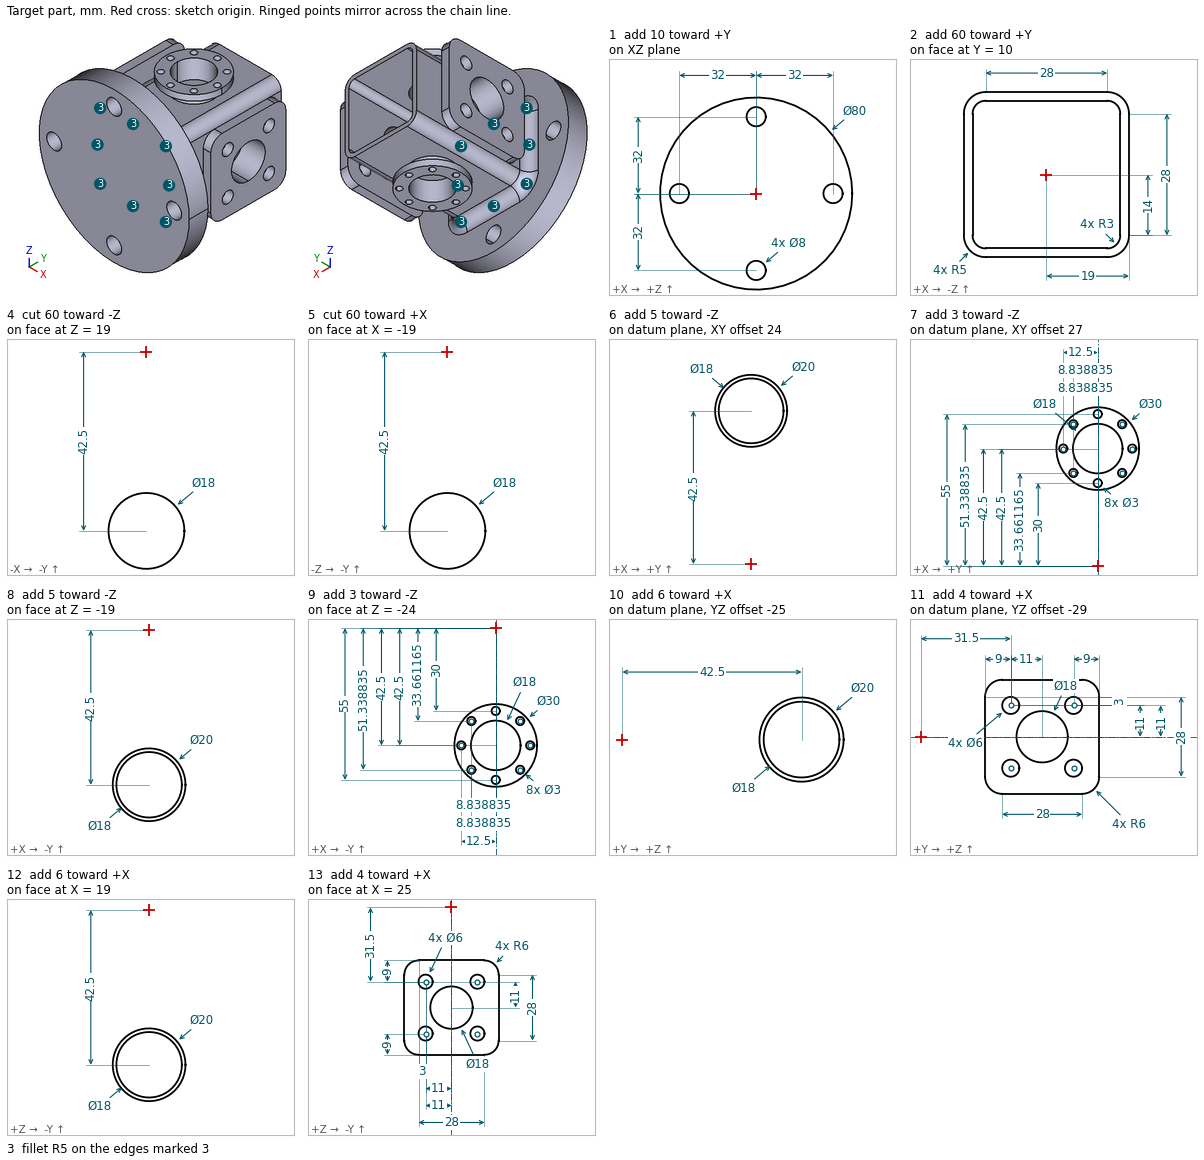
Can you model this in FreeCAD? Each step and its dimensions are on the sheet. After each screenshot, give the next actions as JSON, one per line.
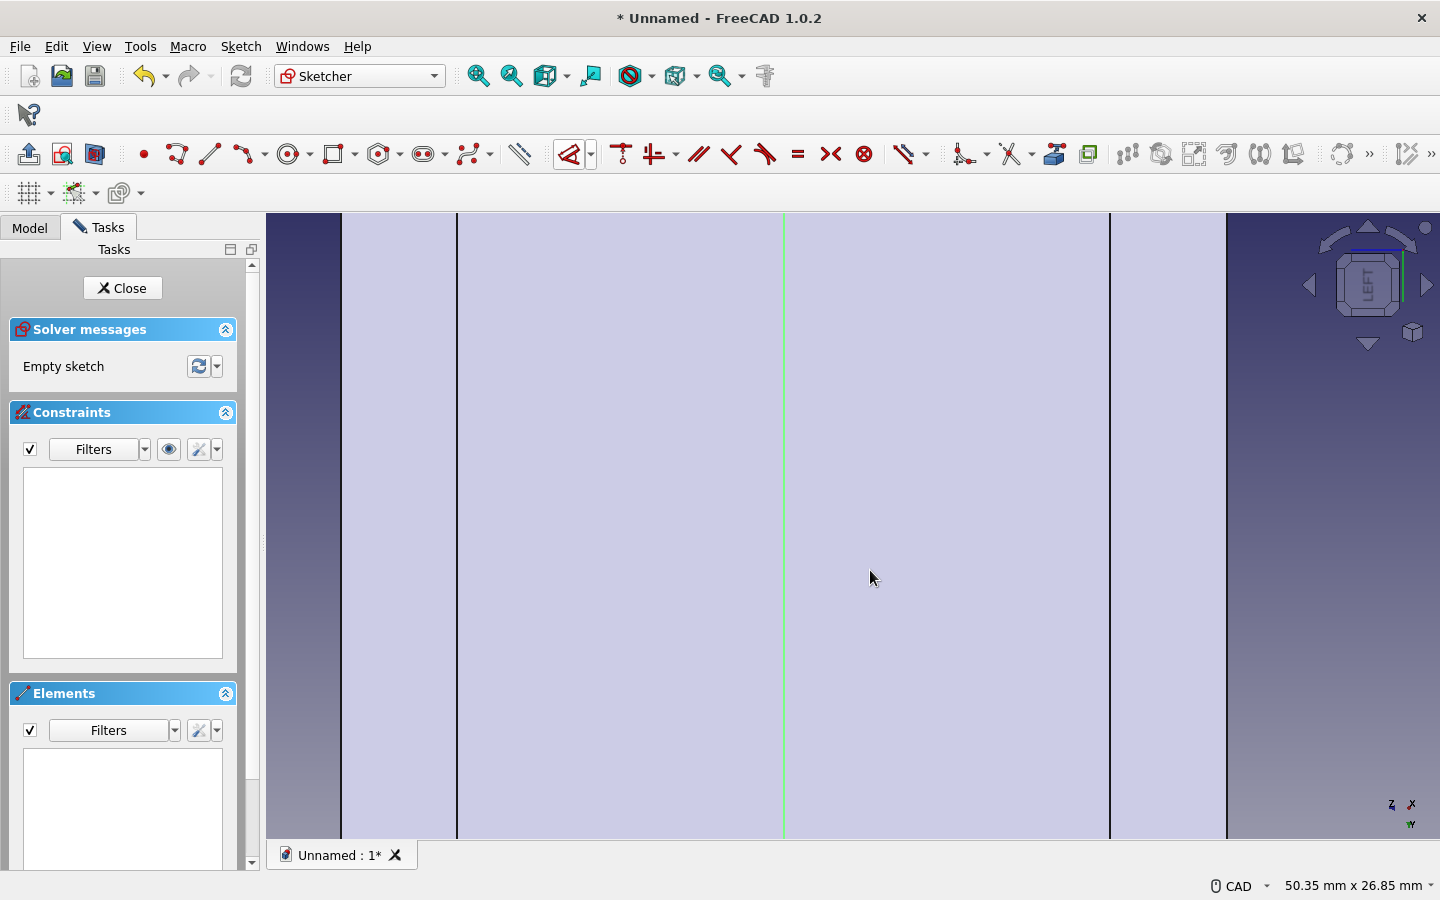
{"action": "key", "text": "g c"}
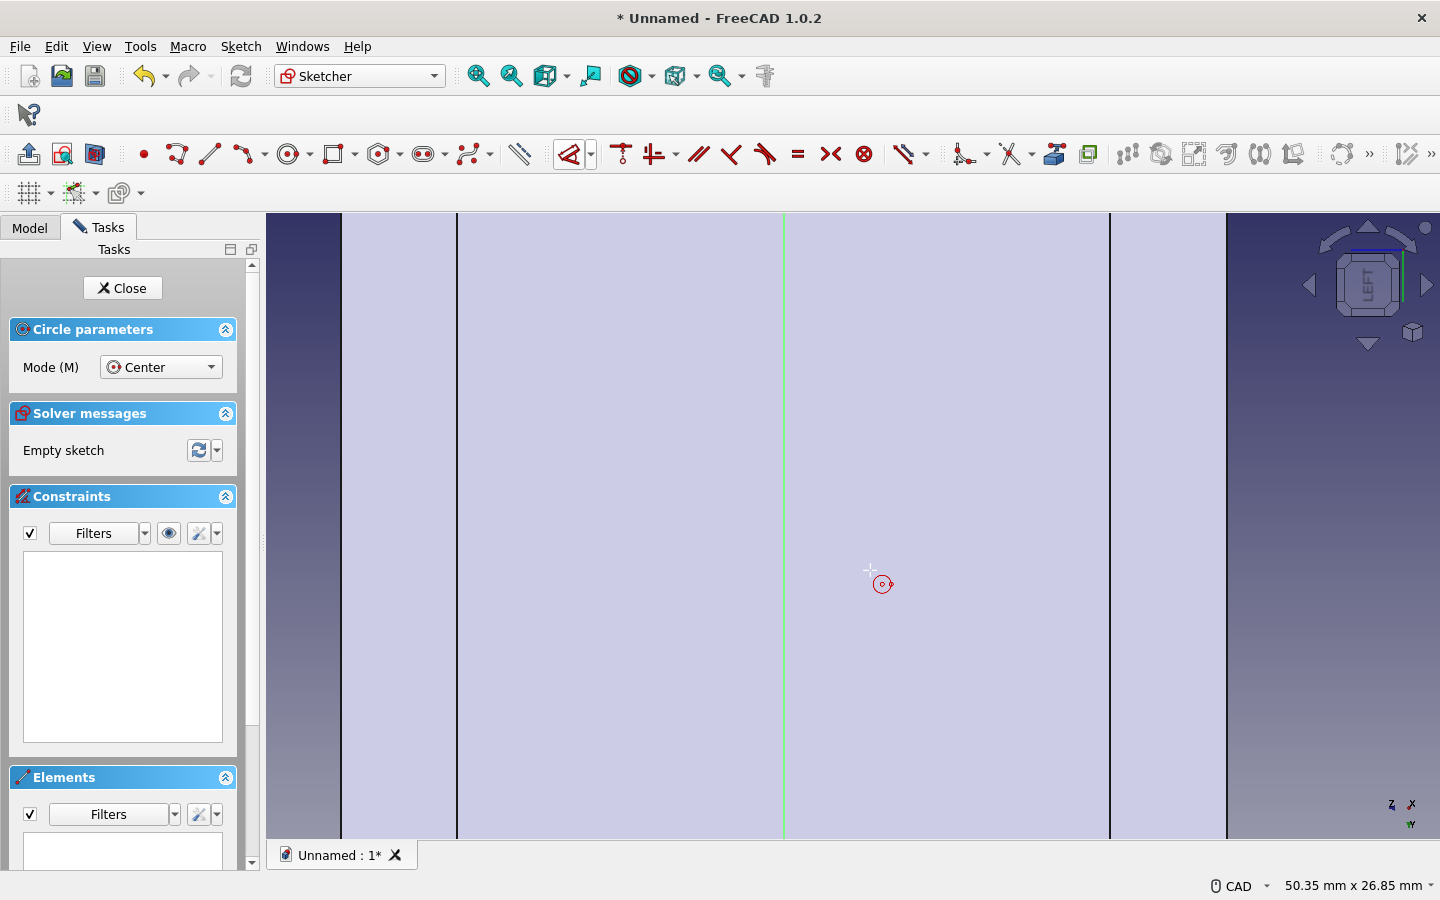
{"action": "left_click", "coordinate": [784, 525]}
{"action": "mouse_move", "coordinate": [932, 376]}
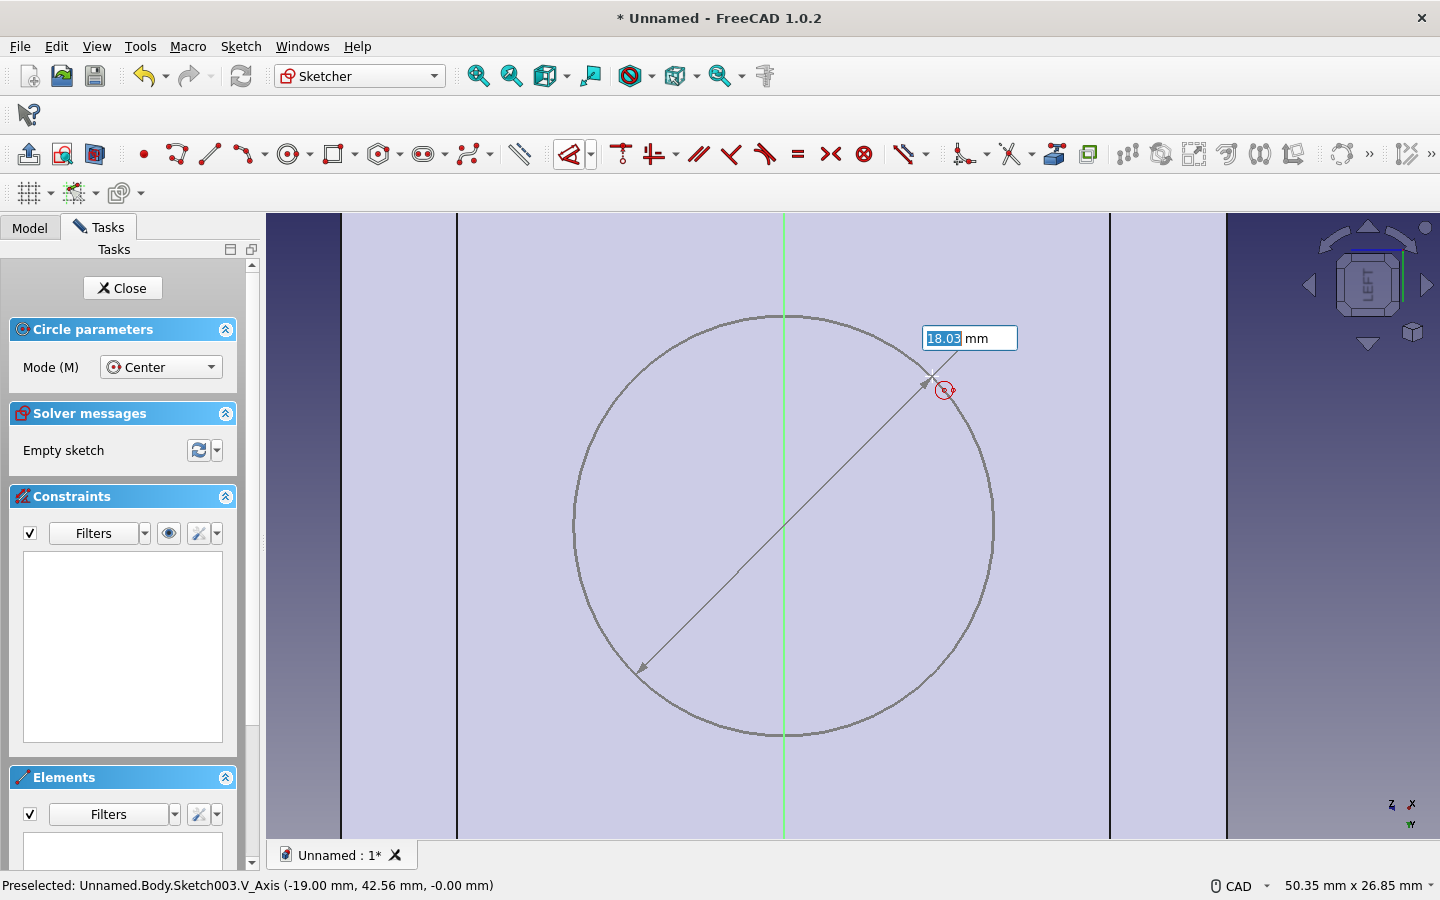
{"action": "type", "text": "18"}
{"action": "key", "text": "Return"}
{"action": "key", "text": "Escape"}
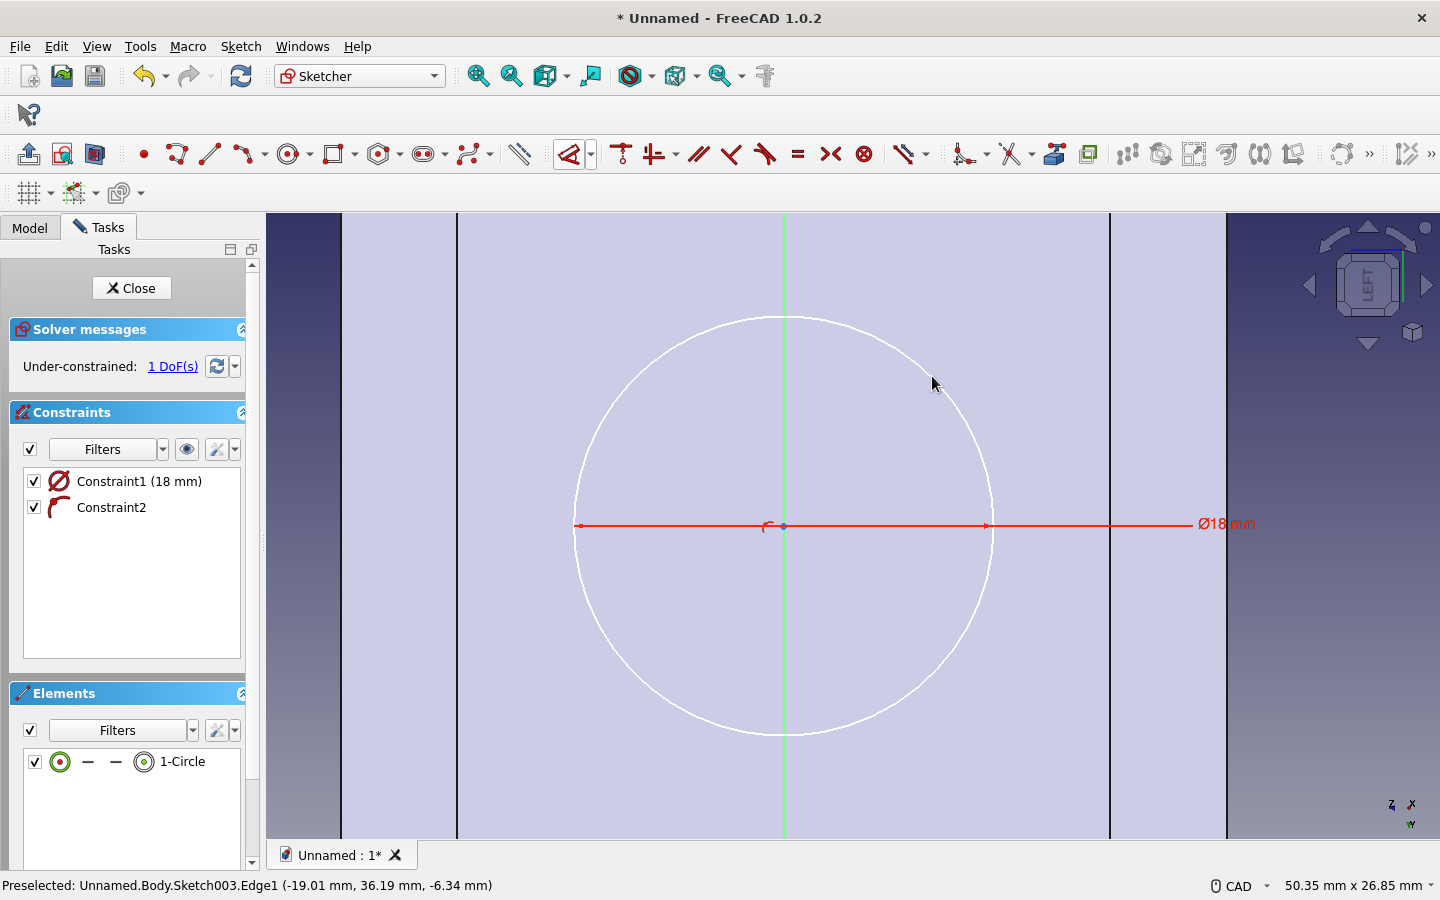
{"action": "left_click", "coordinate": [784, 526]}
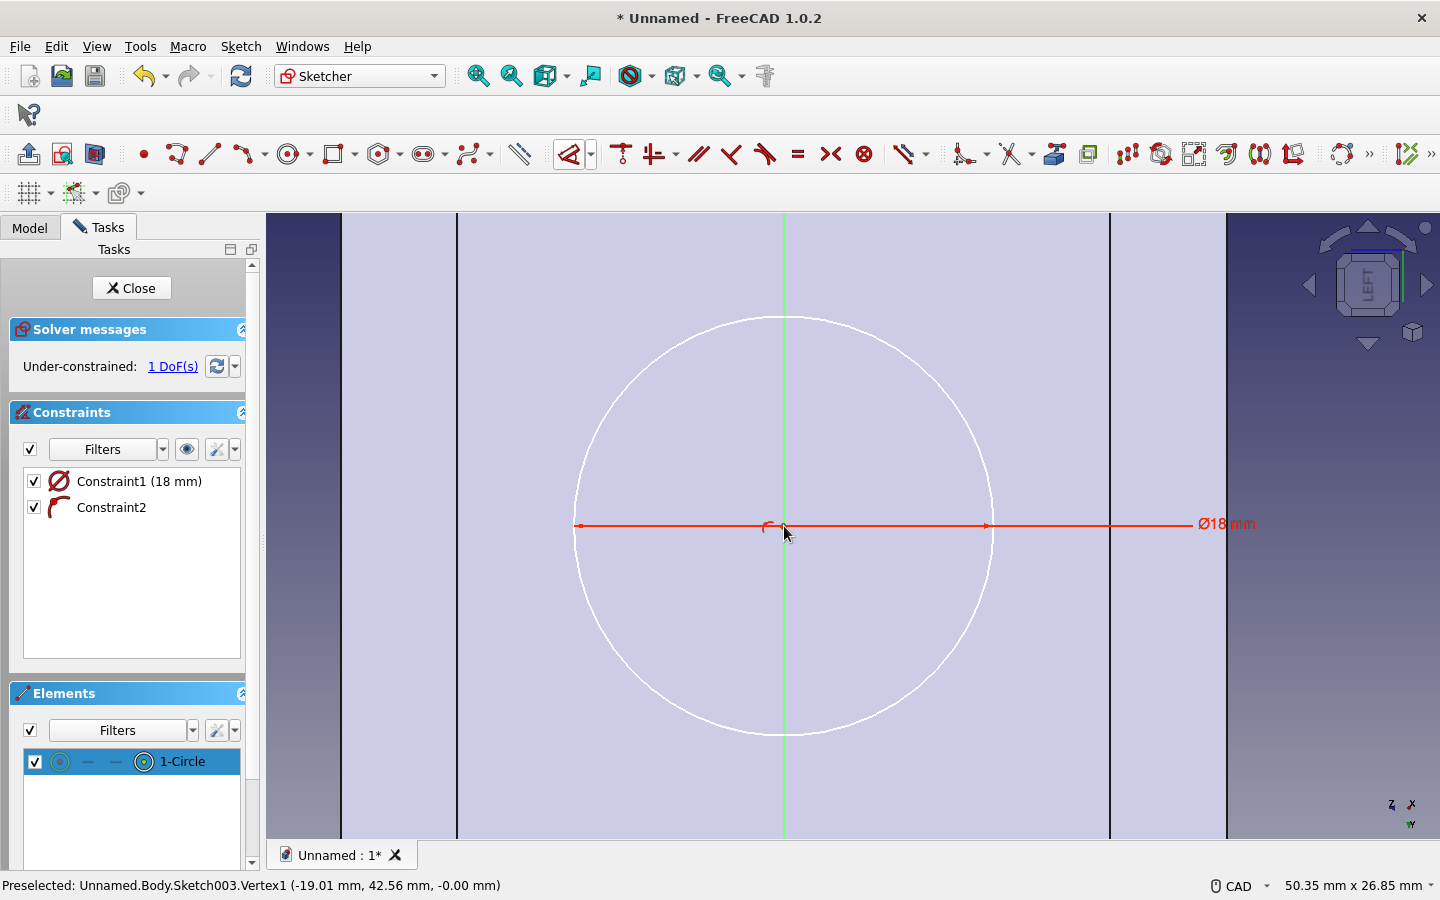
{"action": "left_click", "coordinate": [590, 154]}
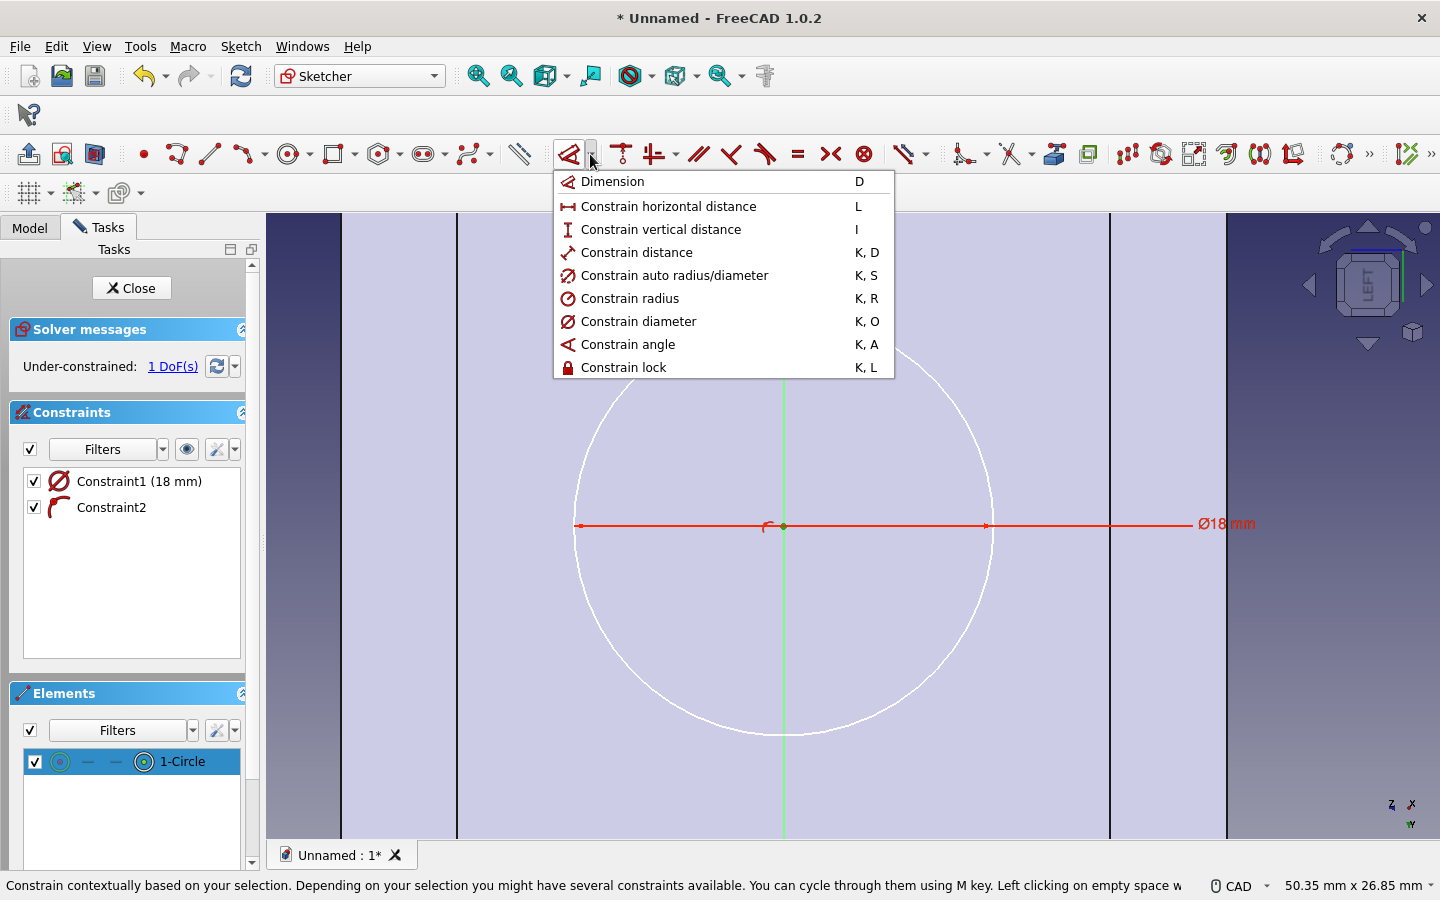
{"action": "left_click", "coordinate": [724, 230]}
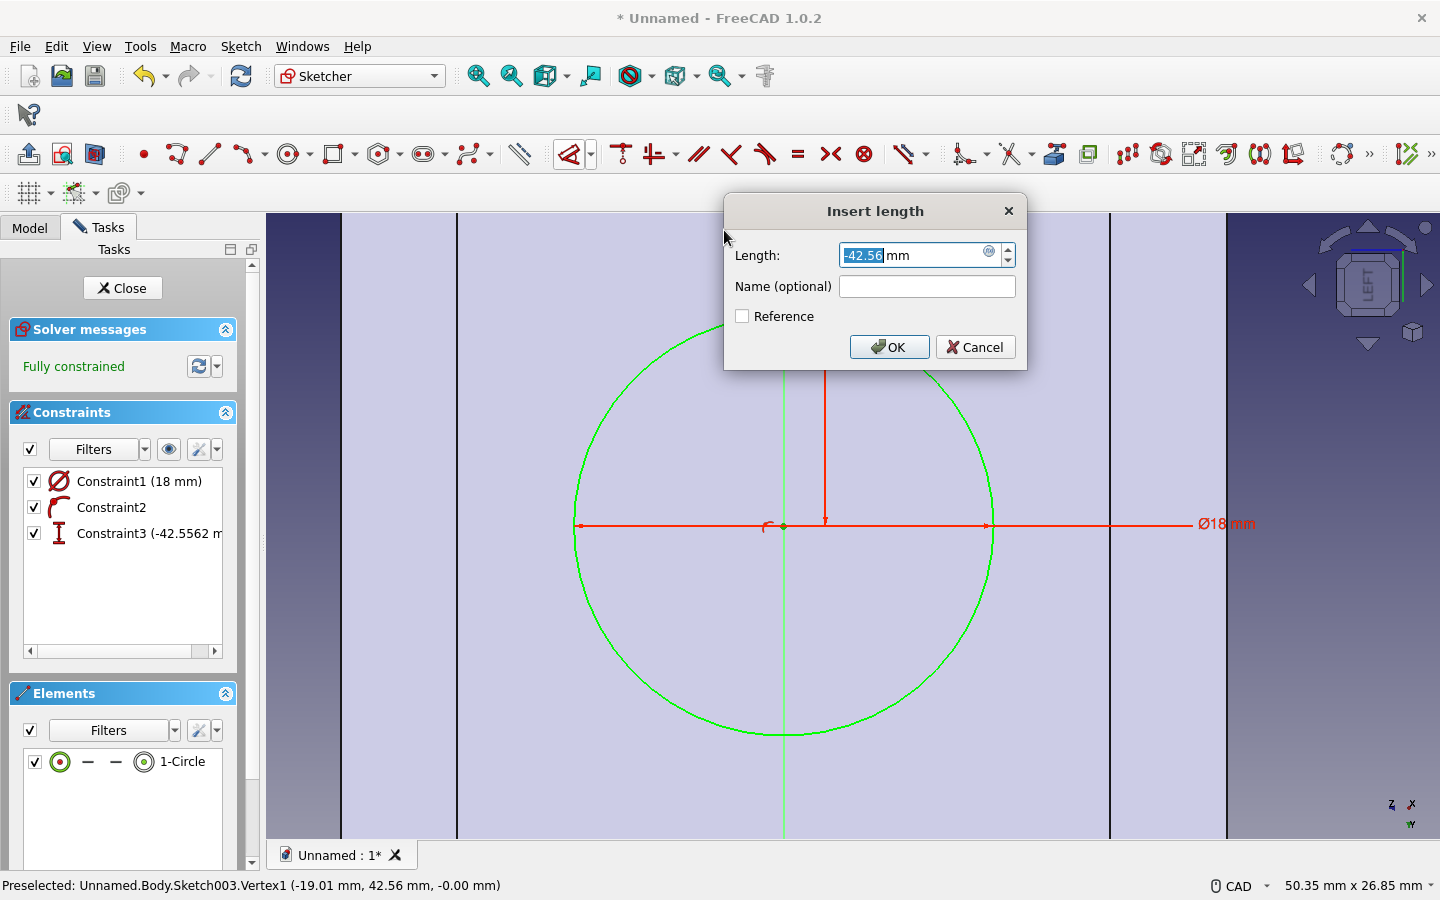
{"action": "type", "text": "-42.5"}
{"action": "key", "text": "Return"}